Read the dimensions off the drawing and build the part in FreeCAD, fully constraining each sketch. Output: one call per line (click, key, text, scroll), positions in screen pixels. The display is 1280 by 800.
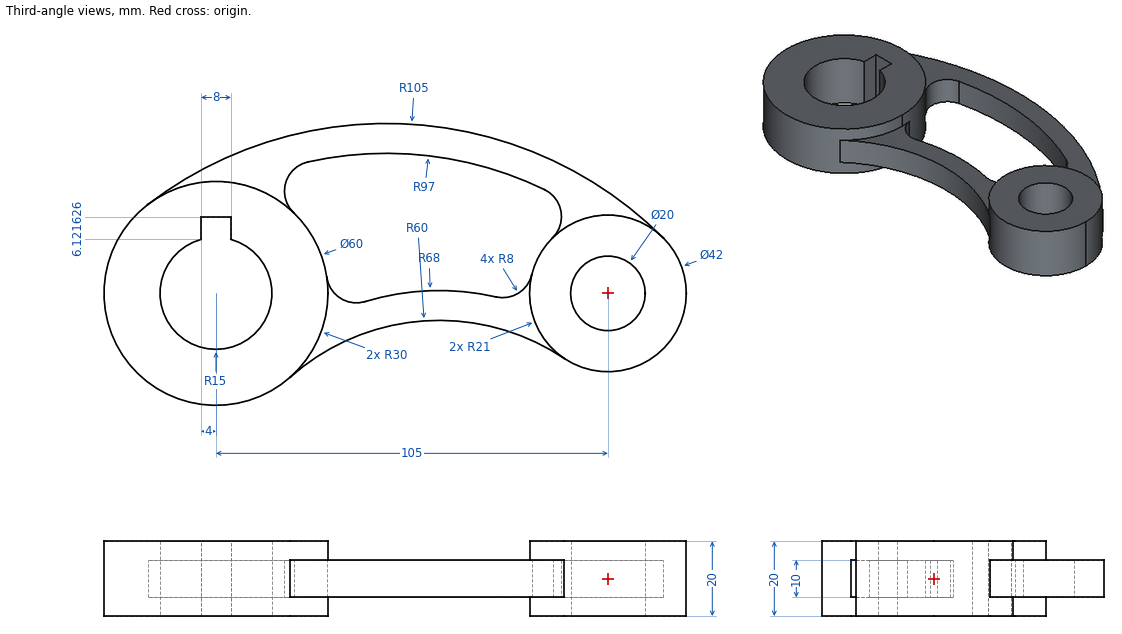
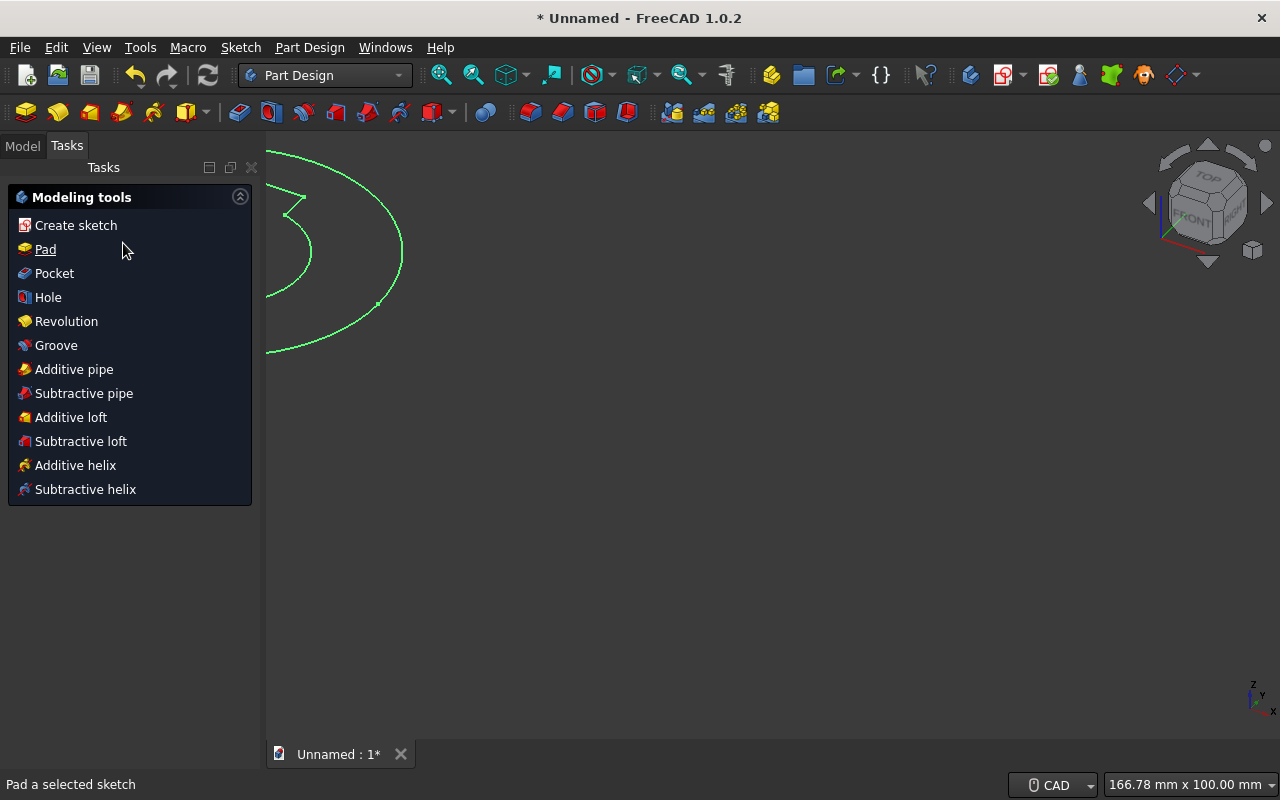
click(26, 112)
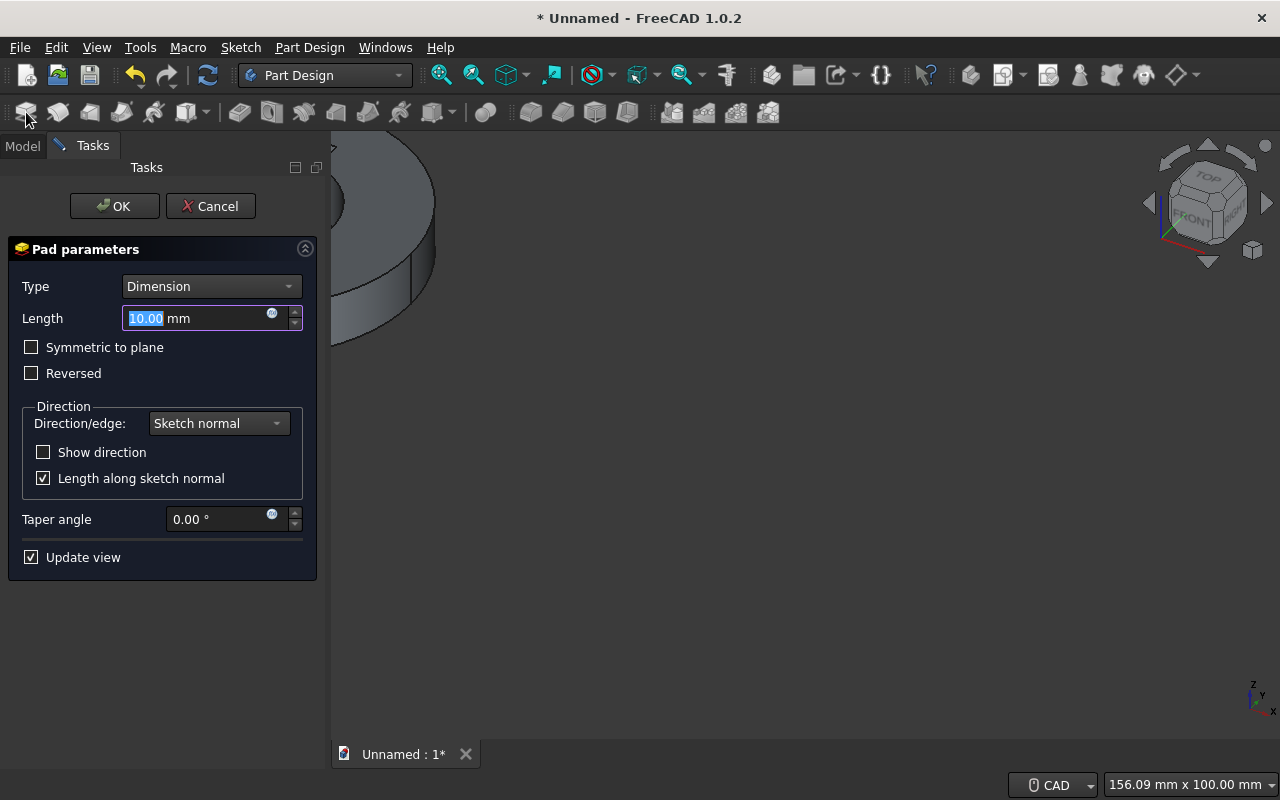
text(20)
key(Tab)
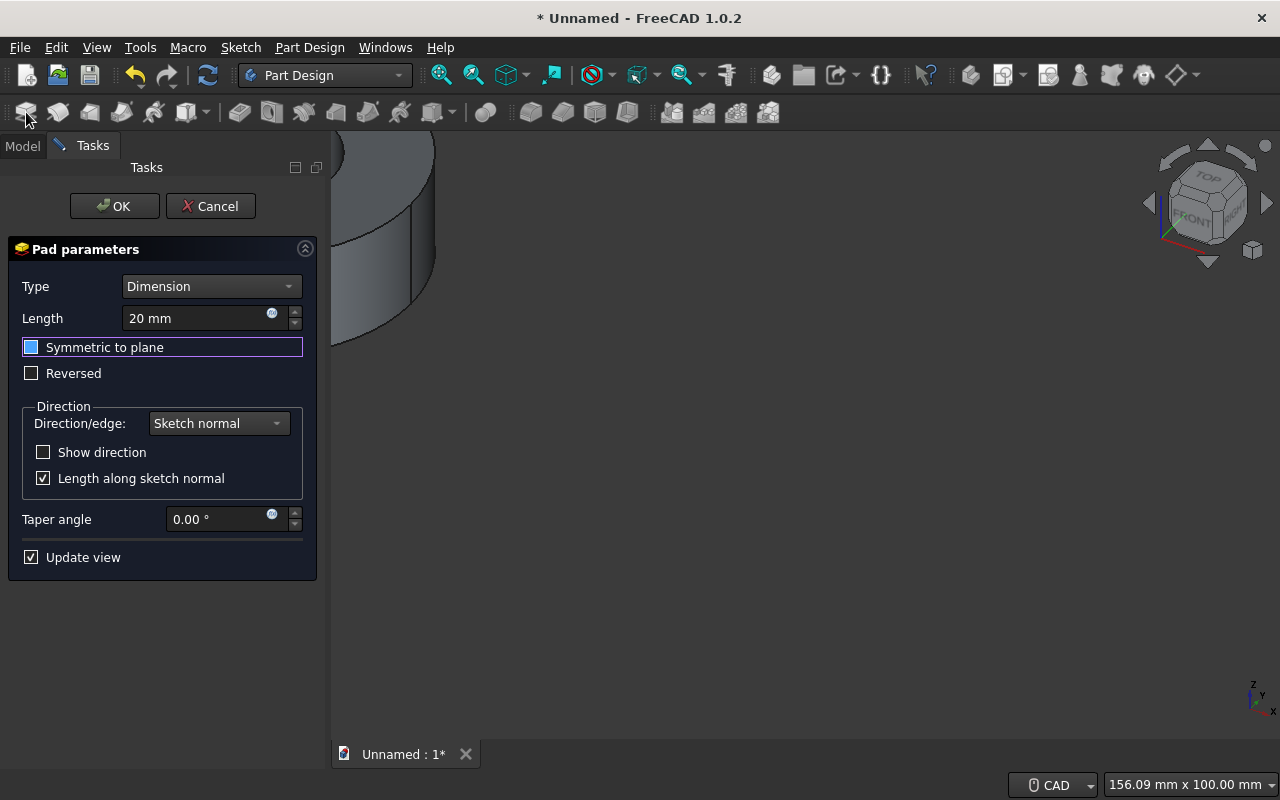
click(30, 347)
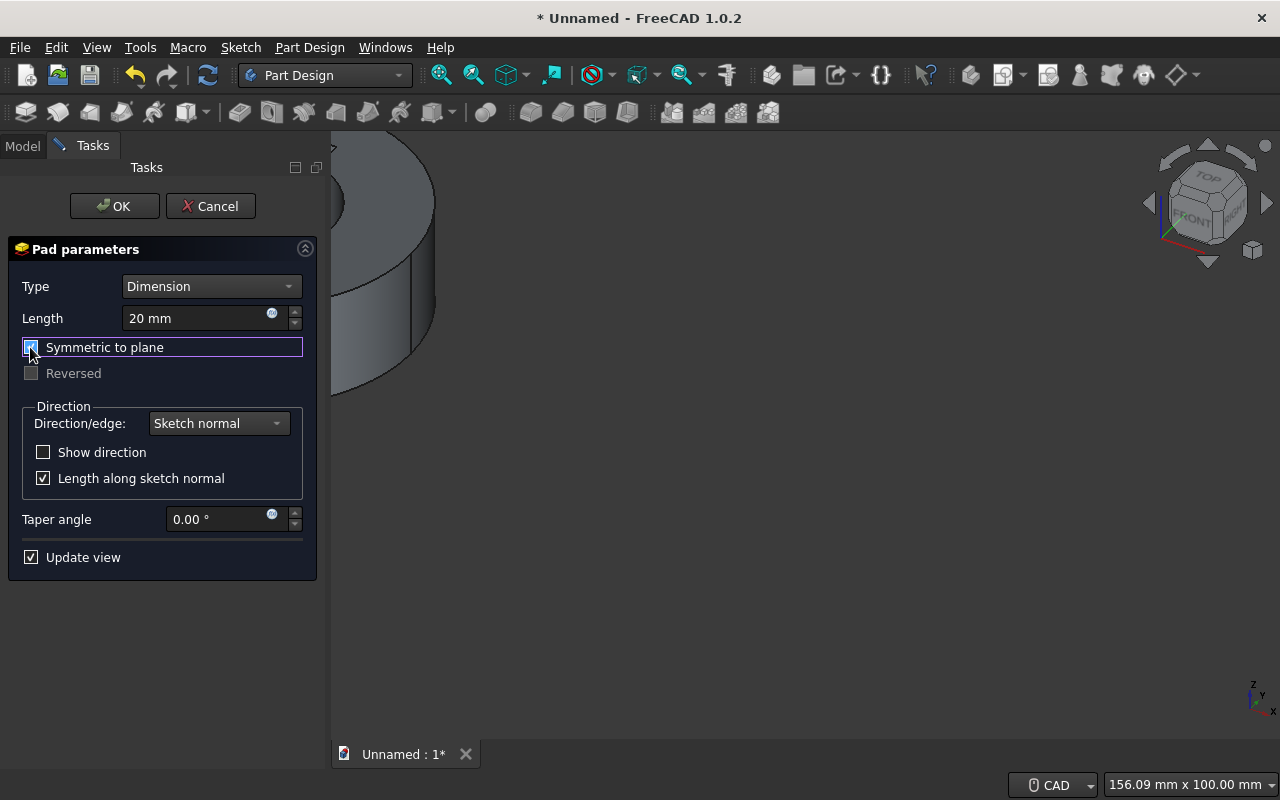
click(115, 206)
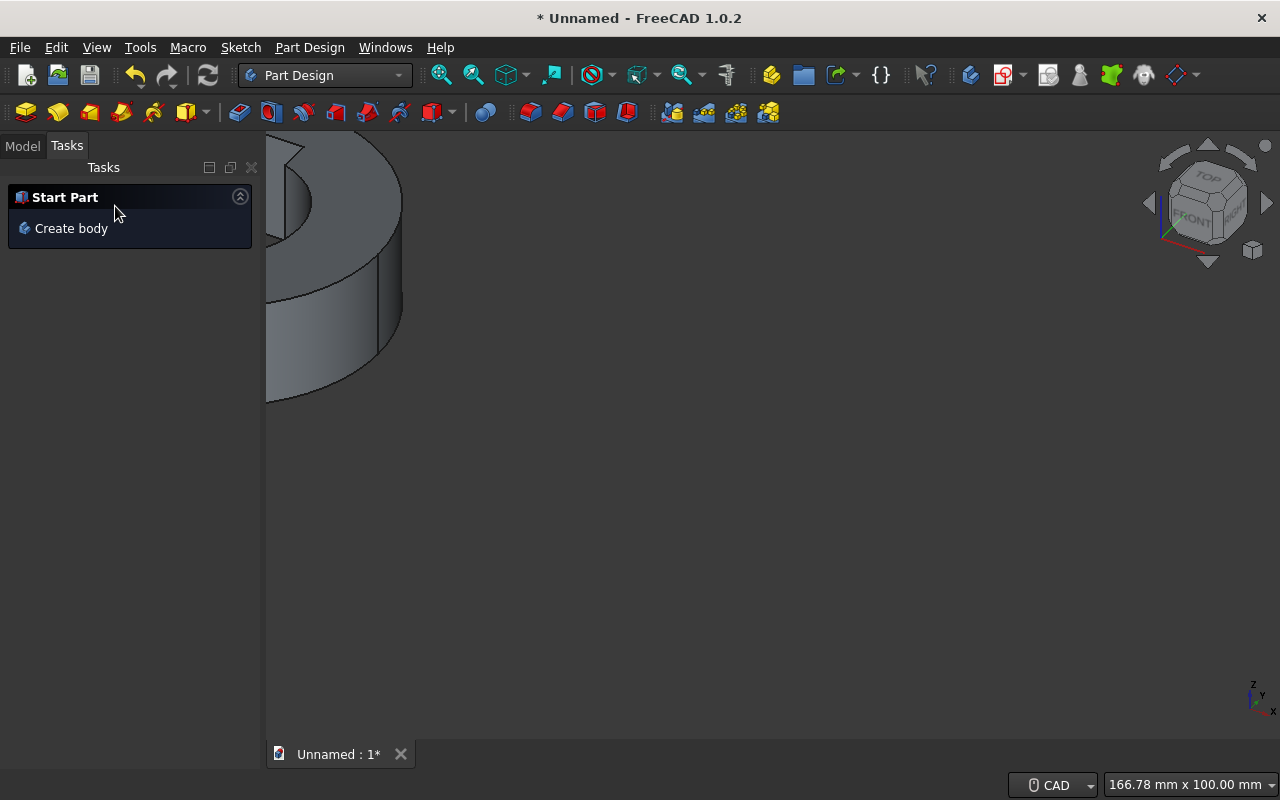
key(v)
key(f)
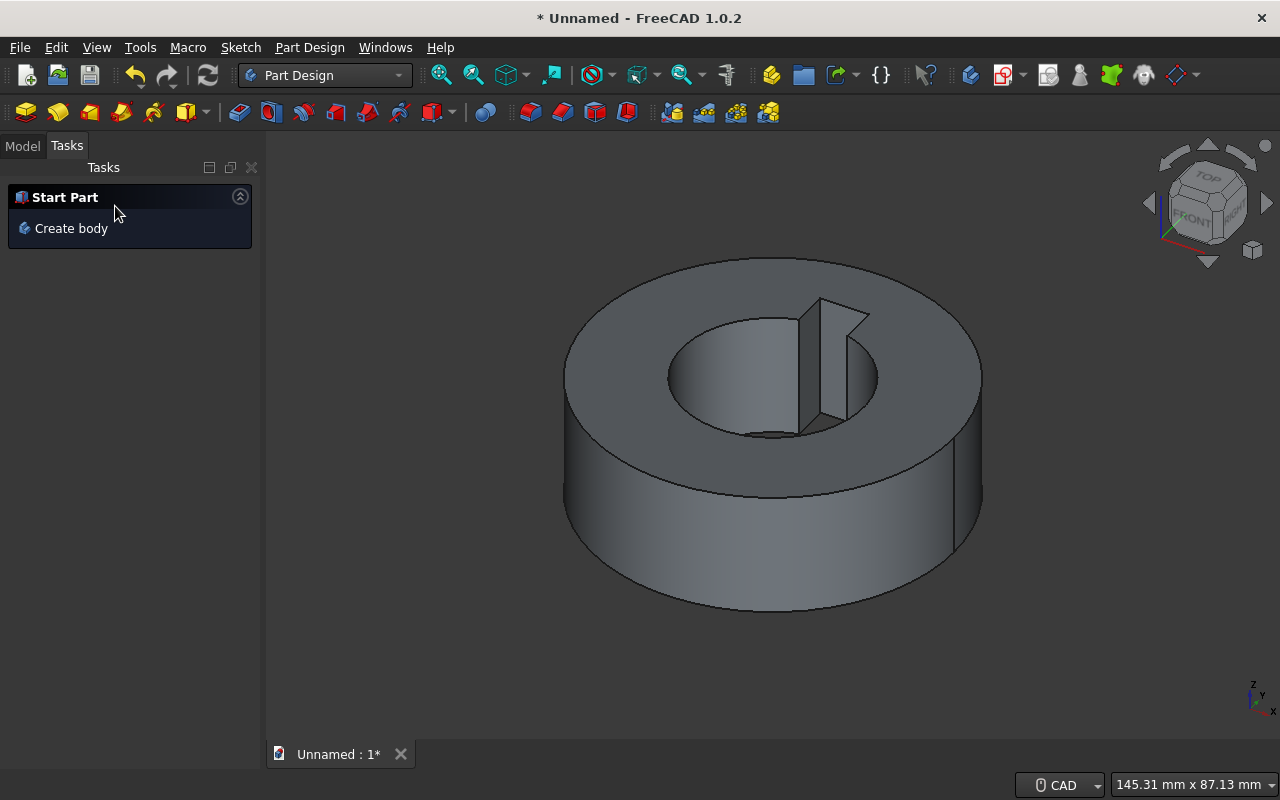
click(972, 76)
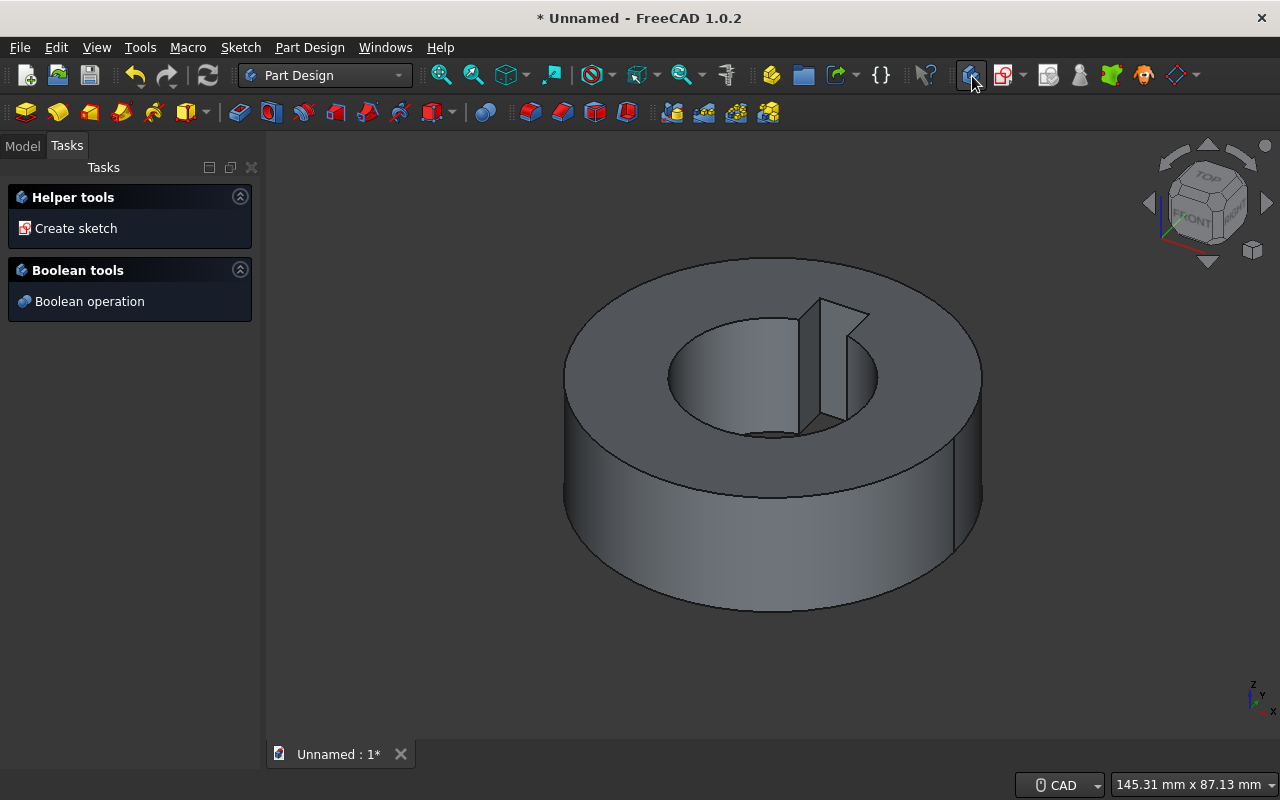
click(306, 699)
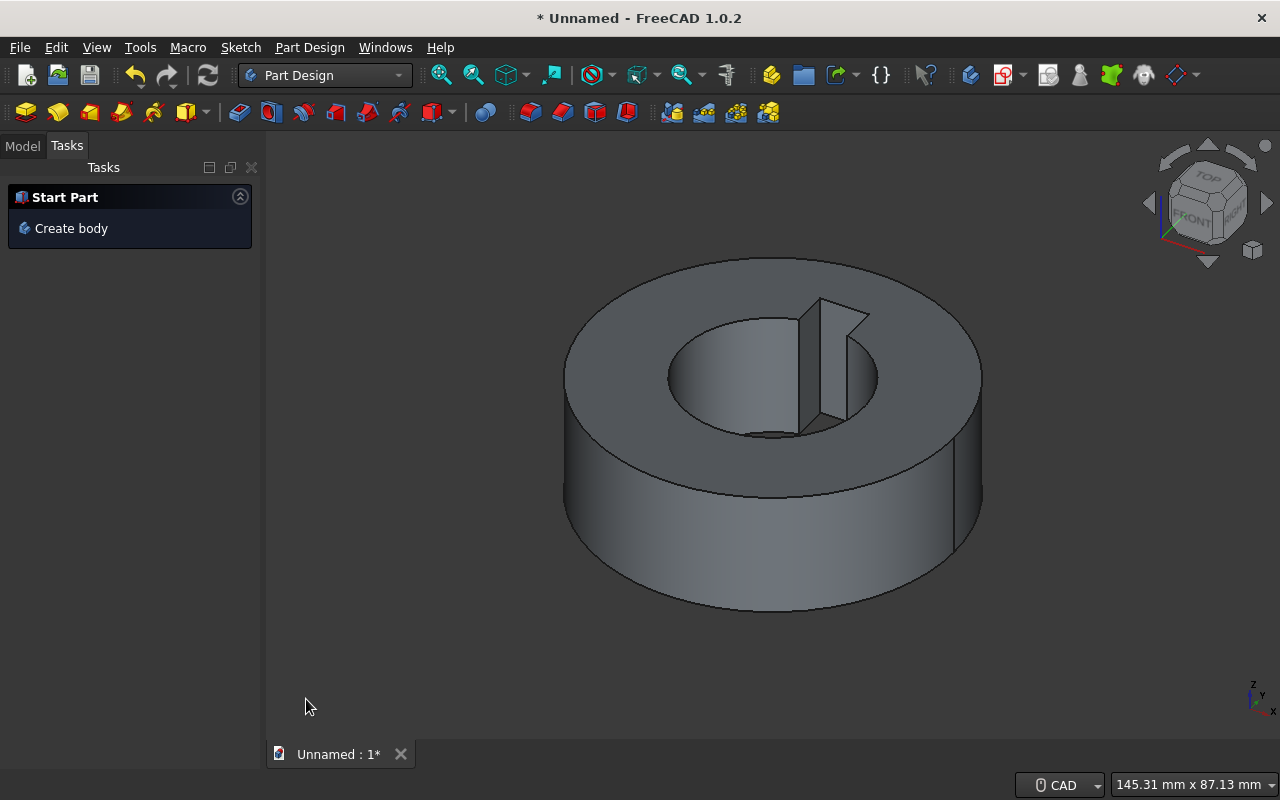
click(1004, 76)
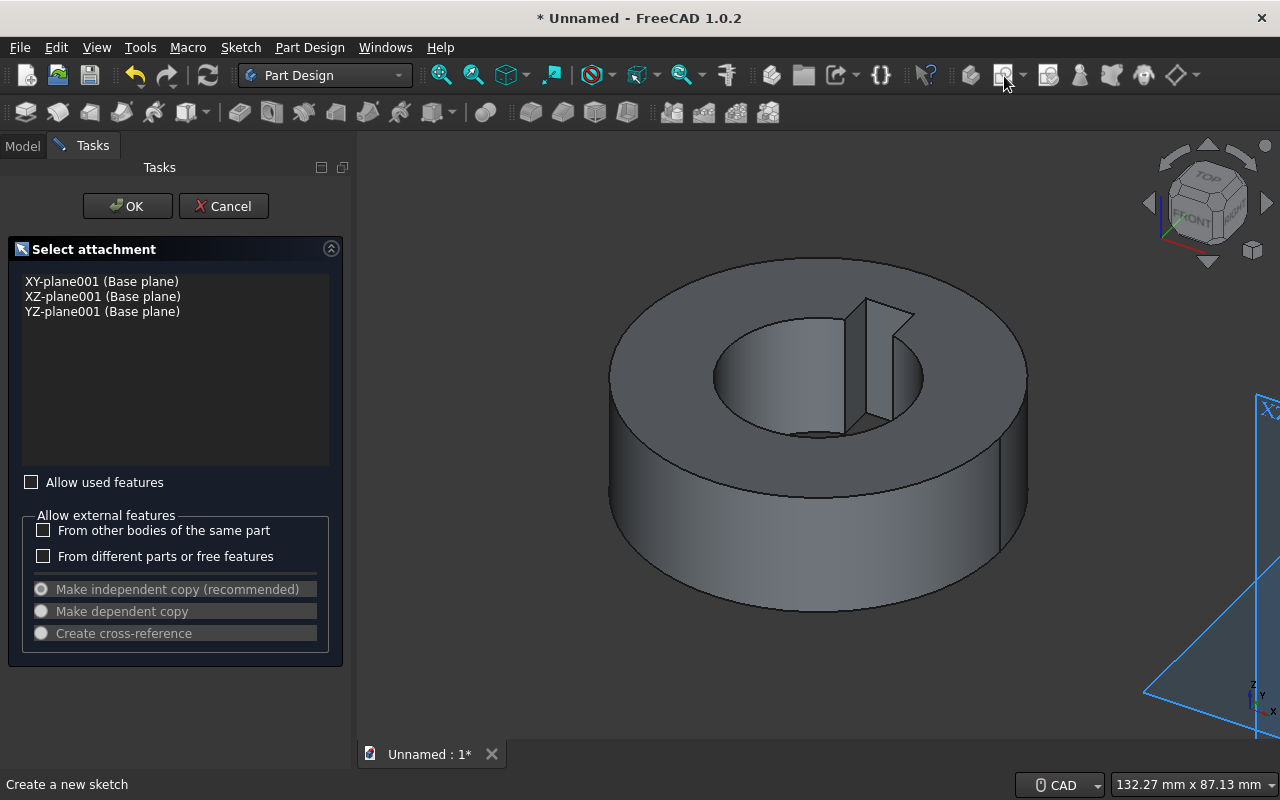
click(82, 282)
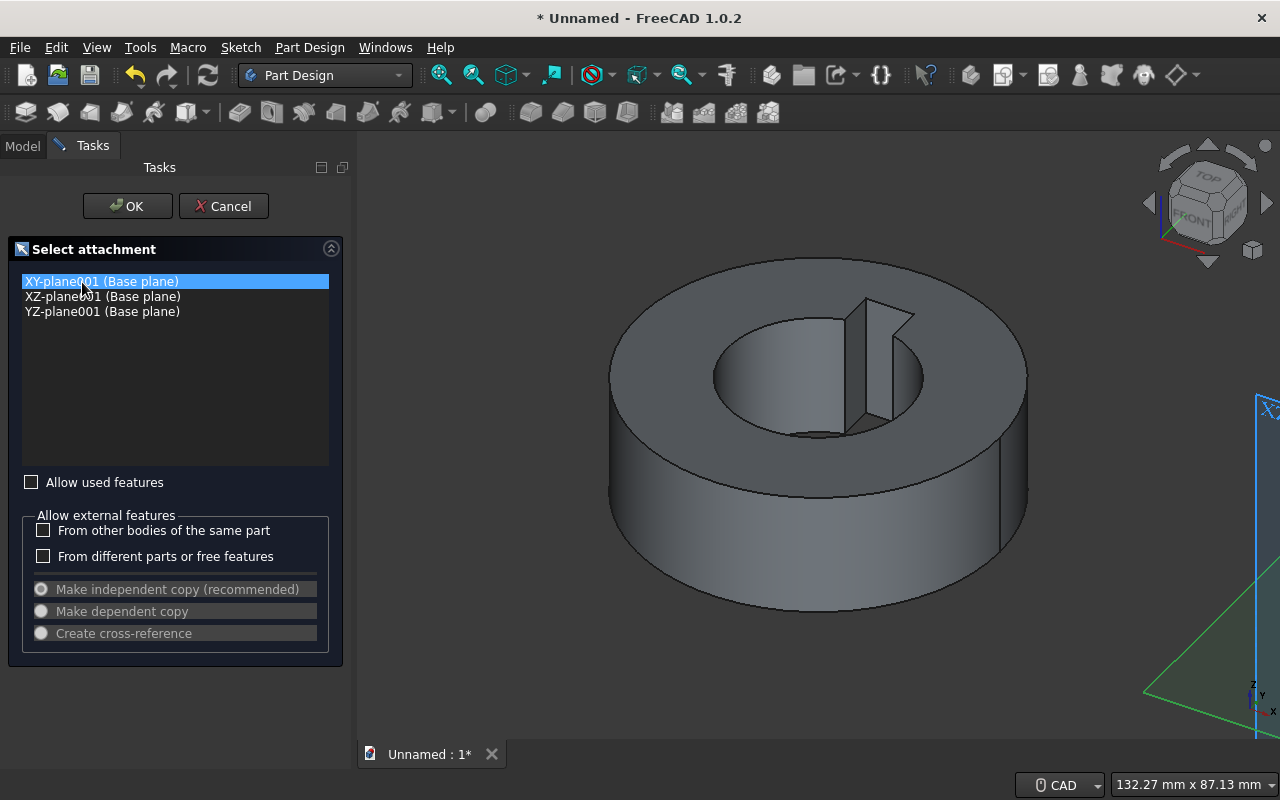
click(128, 206)